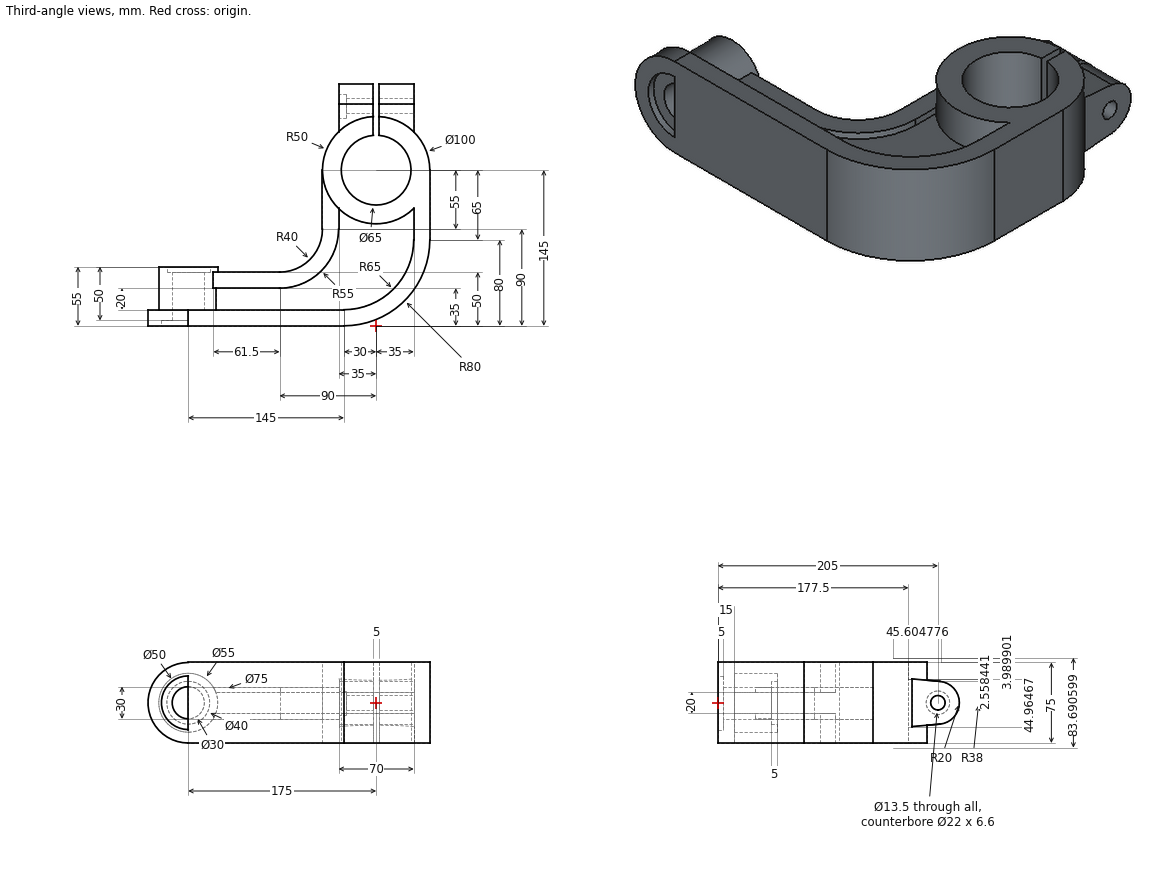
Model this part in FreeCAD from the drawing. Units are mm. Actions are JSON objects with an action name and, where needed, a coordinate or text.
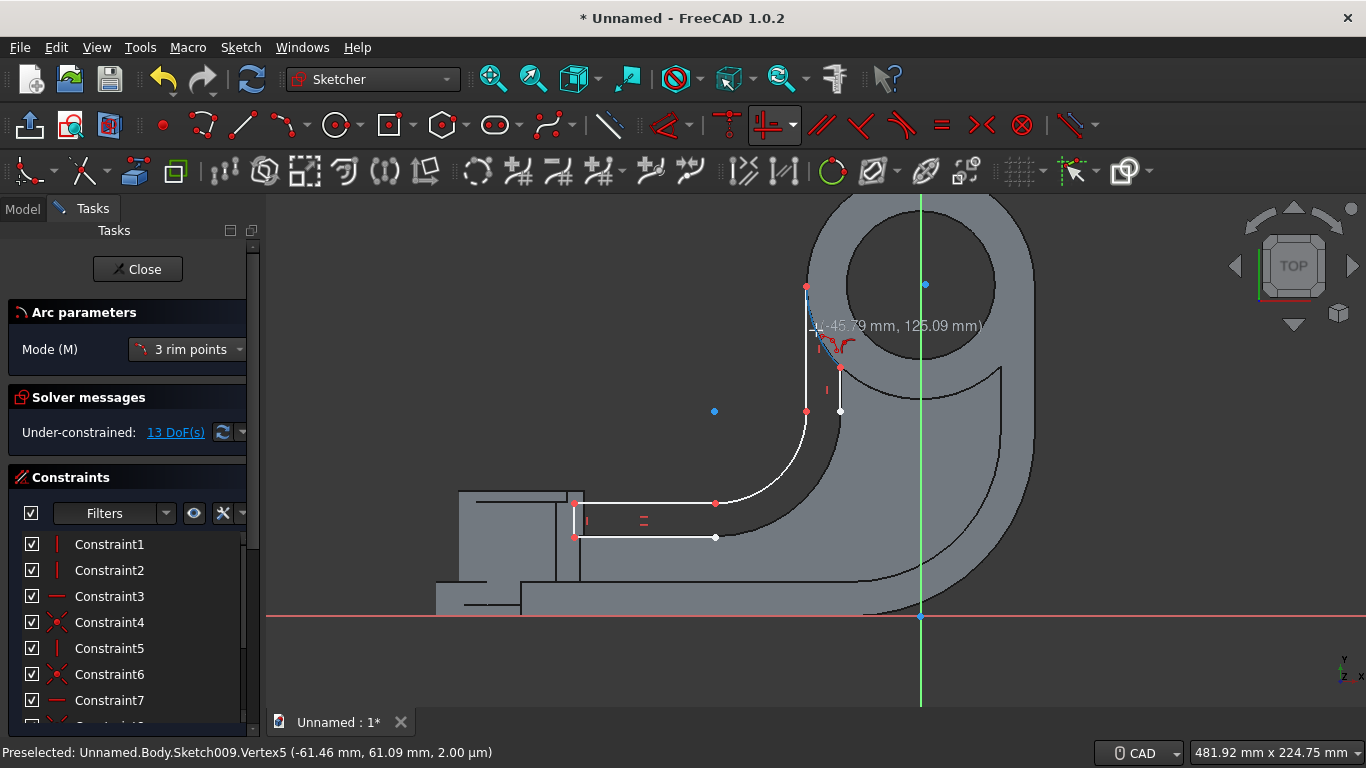
{"action": "left_click", "coordinate": [715, 537]}
{"action": "left_click", "coordinate": [840, 411]}
{"action": "left_click", "coordinate": [804, 500]}
{"action": "key", "text": "Escape"}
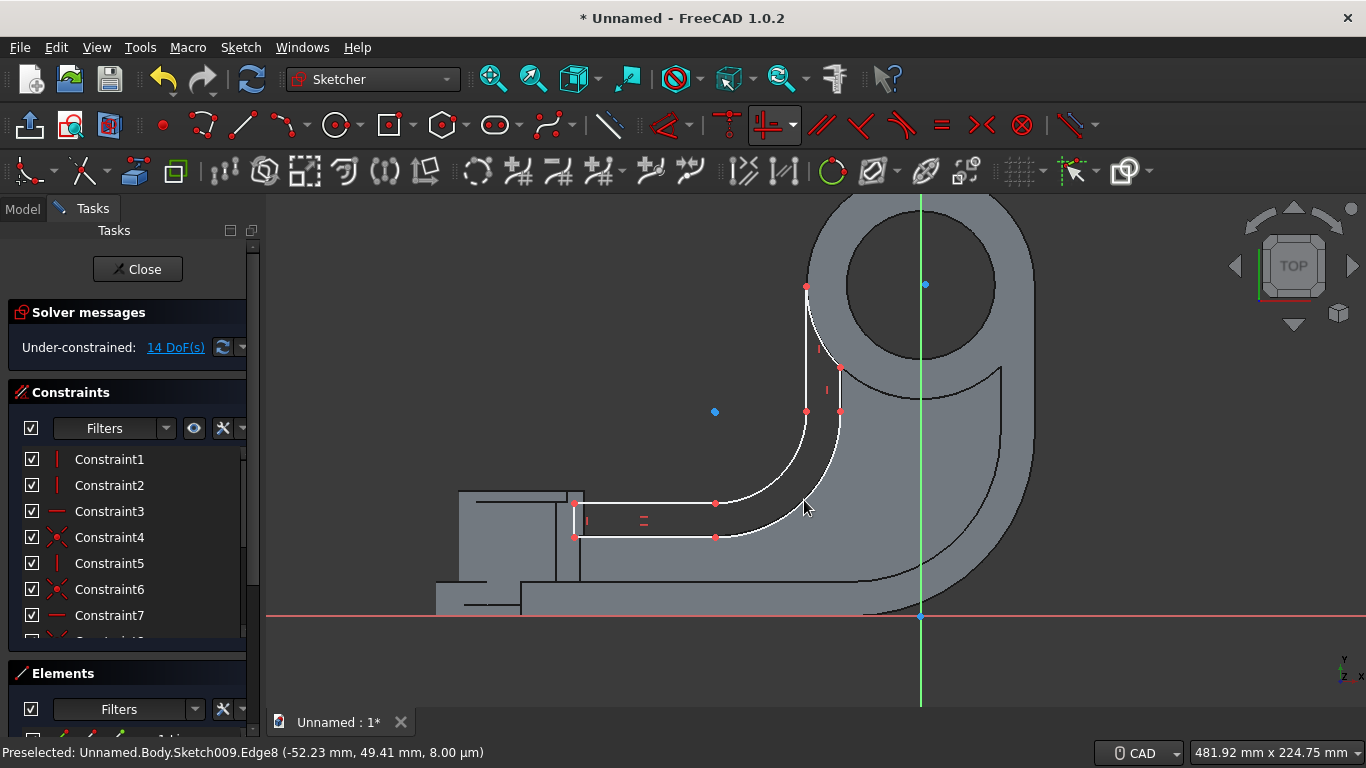
{"action": "left_click", "coordinate": [757, 493]}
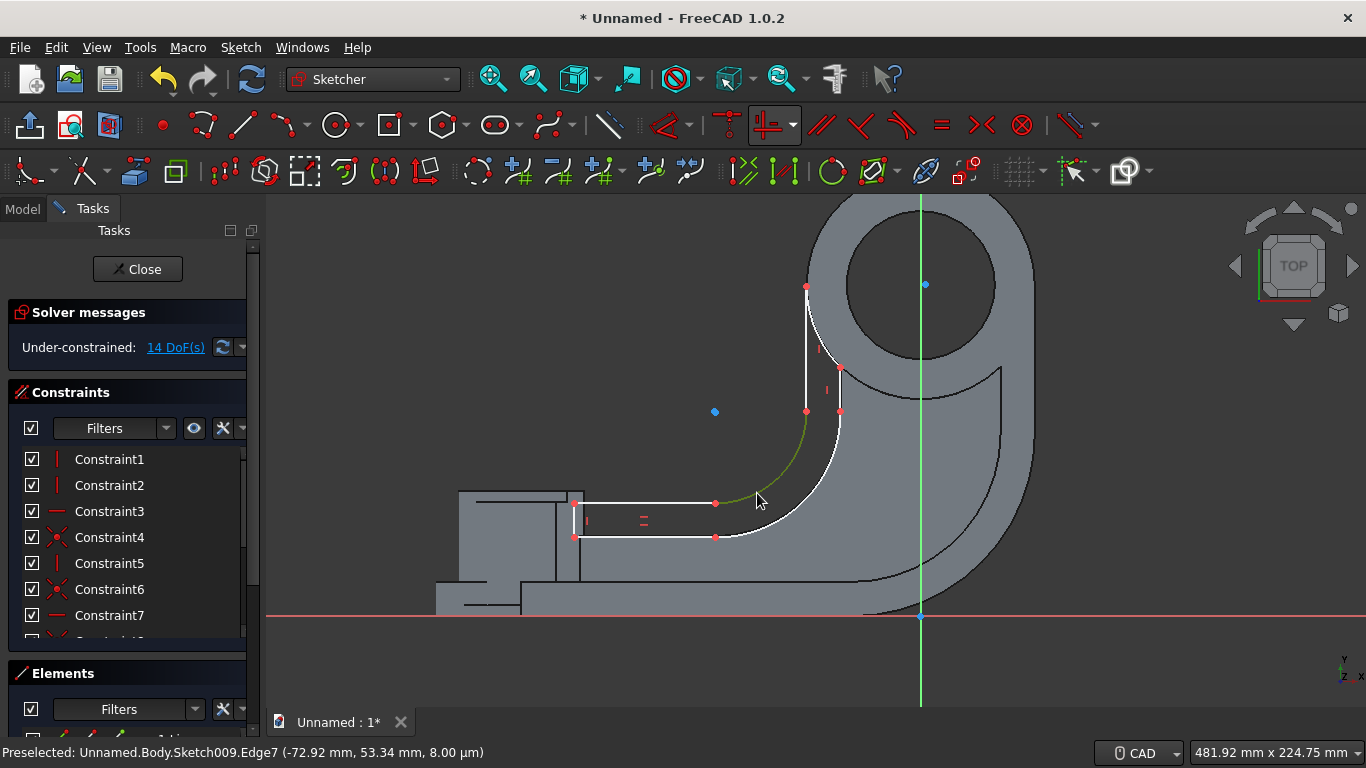
{"action": "left_click", "coordinate": [773, 524]}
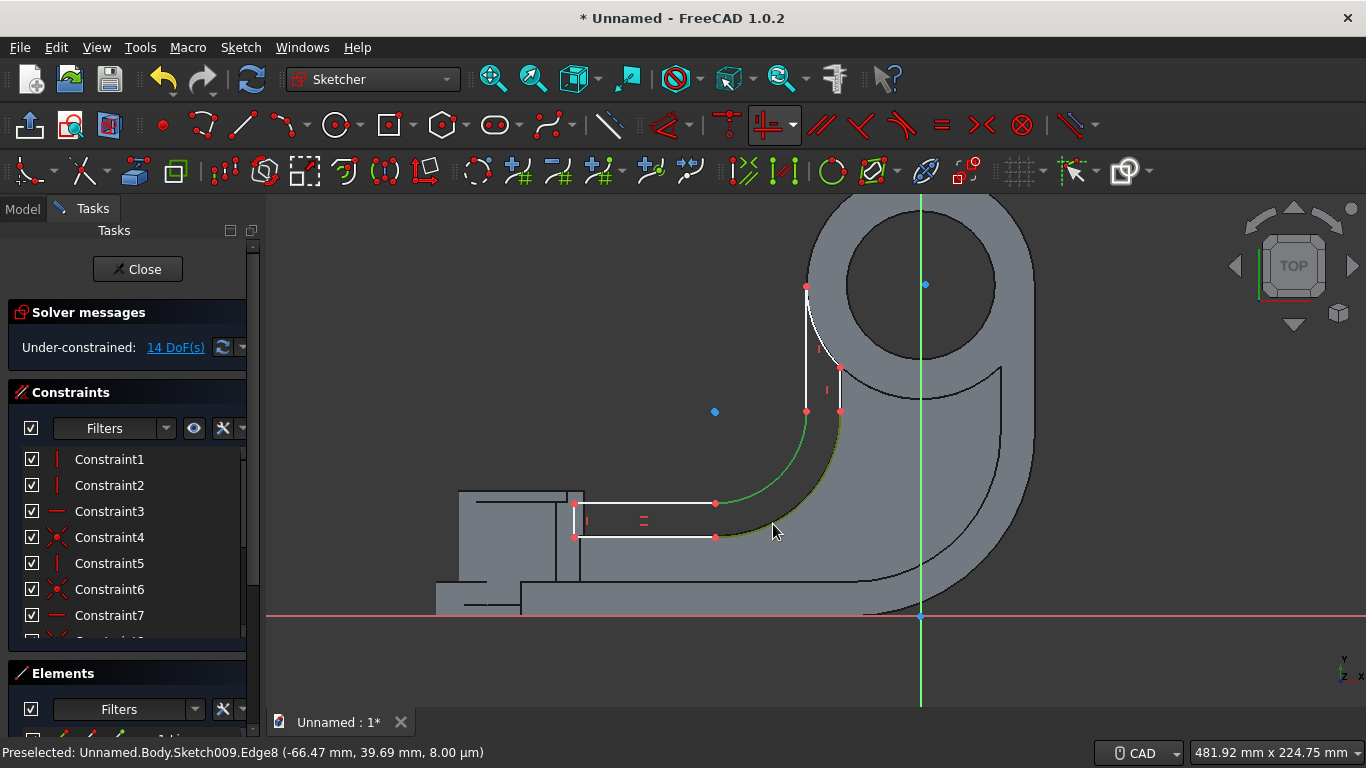
{"action": "left_click", "coordinate": [728, 126]}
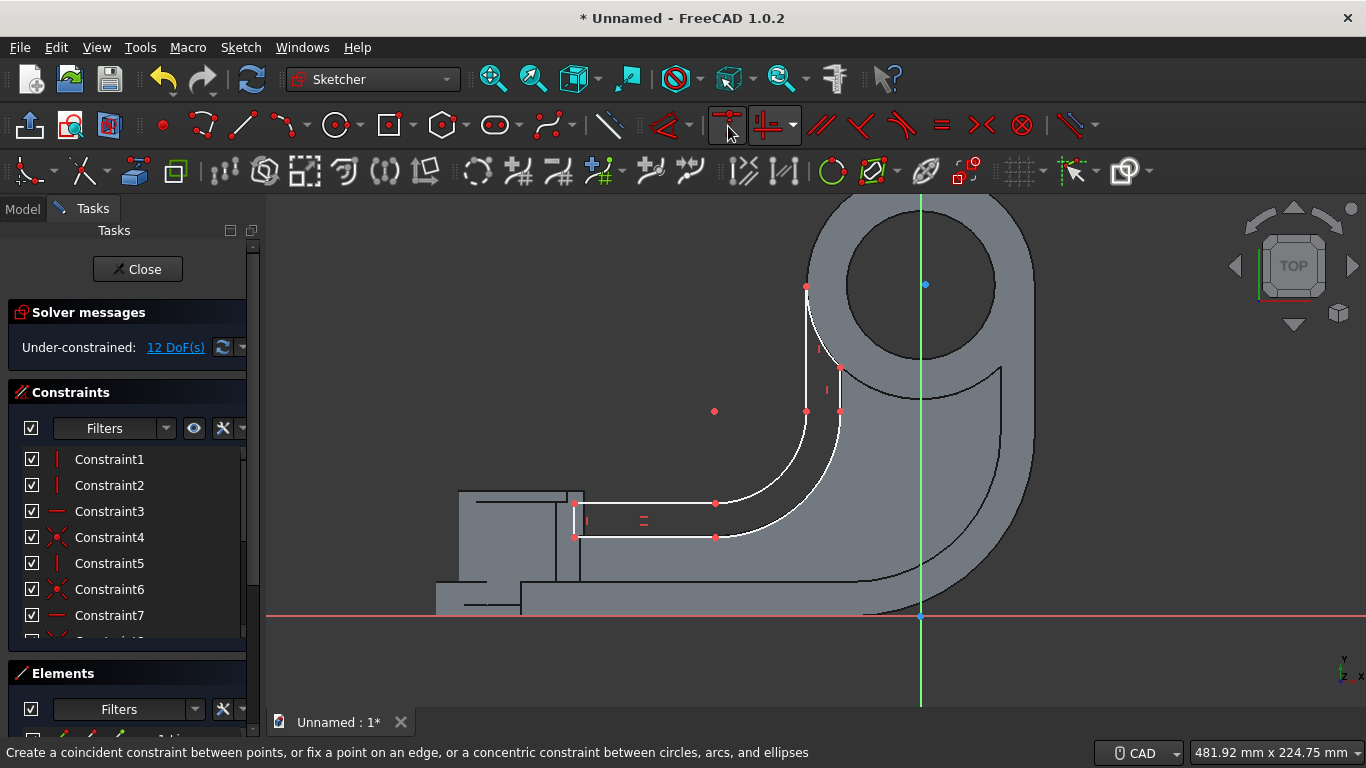
{"action": "left_click", "coordinate": [926, 284]}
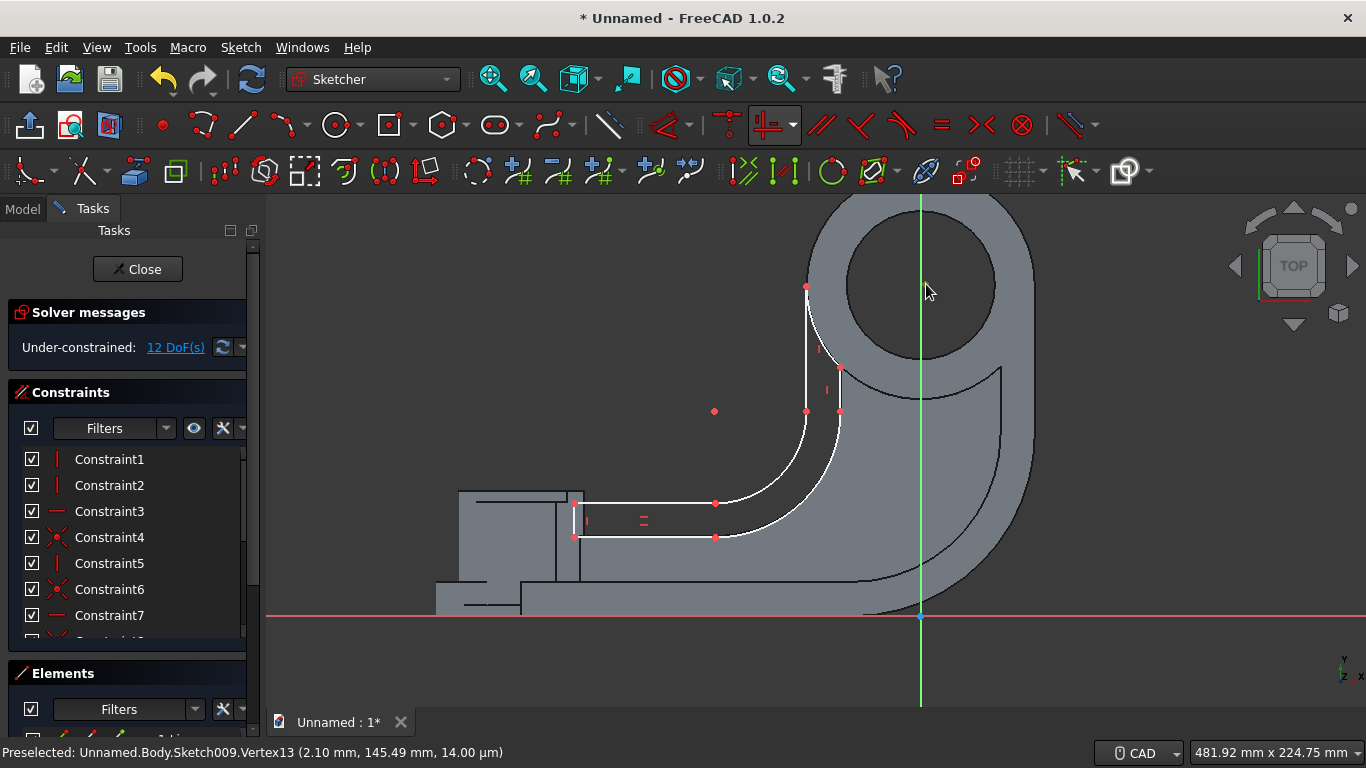
{"action": "left_click", "coordinate": [921, 646]}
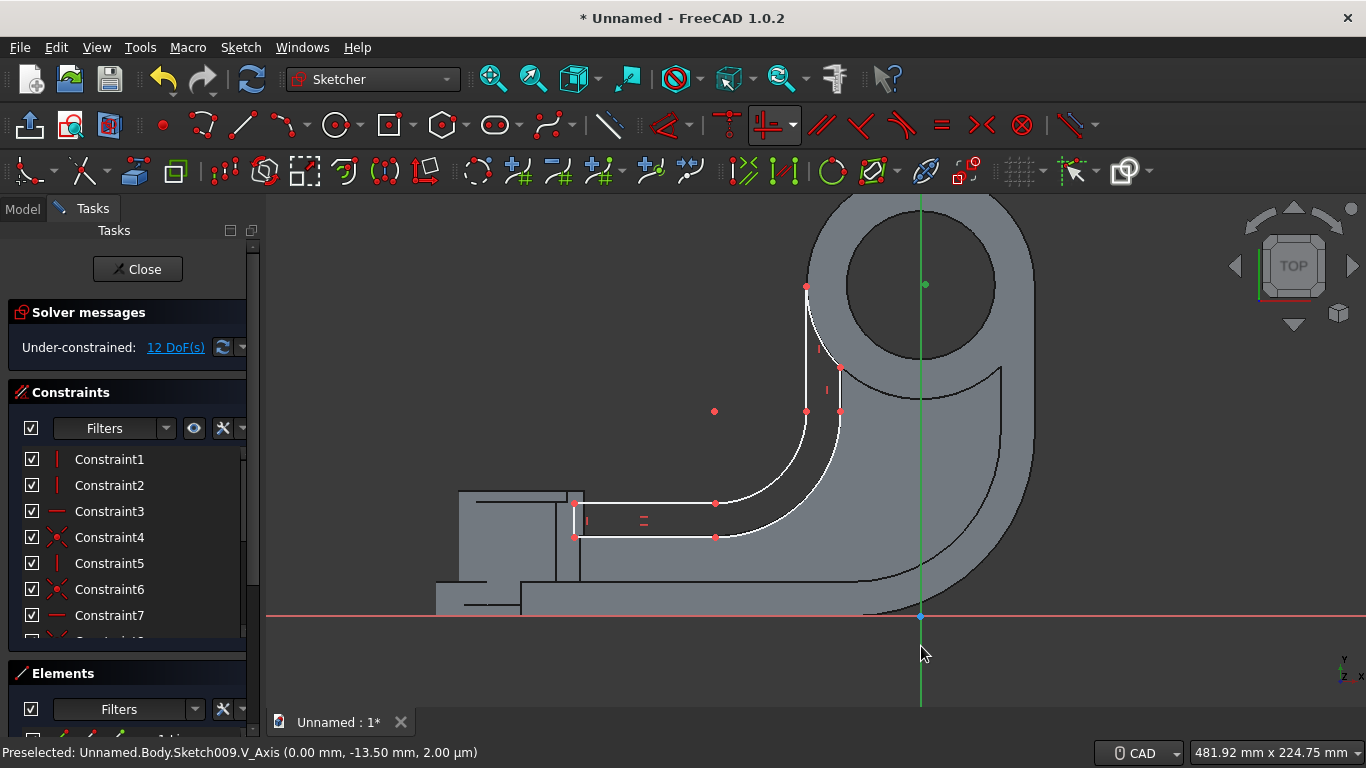
{"action": "key", "text": "c"}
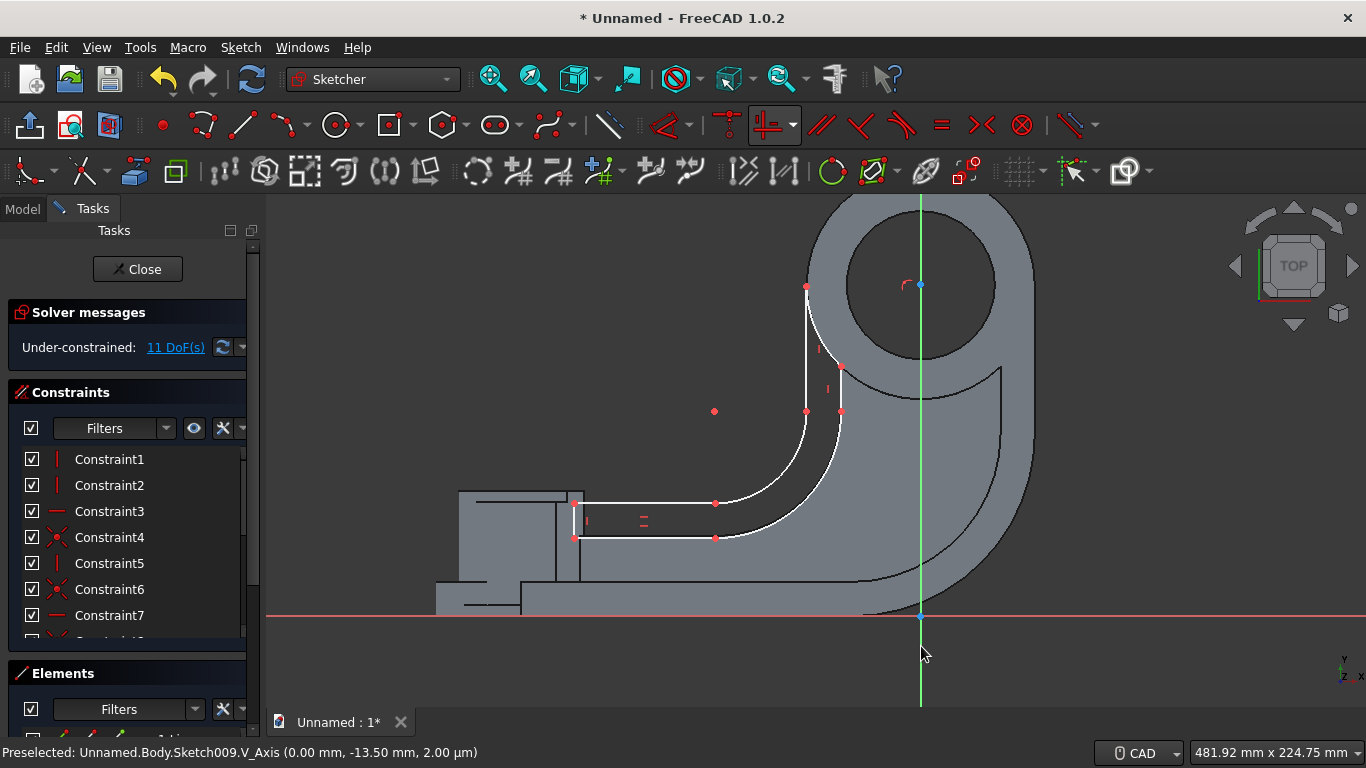
{"action": "key", "text": "d"}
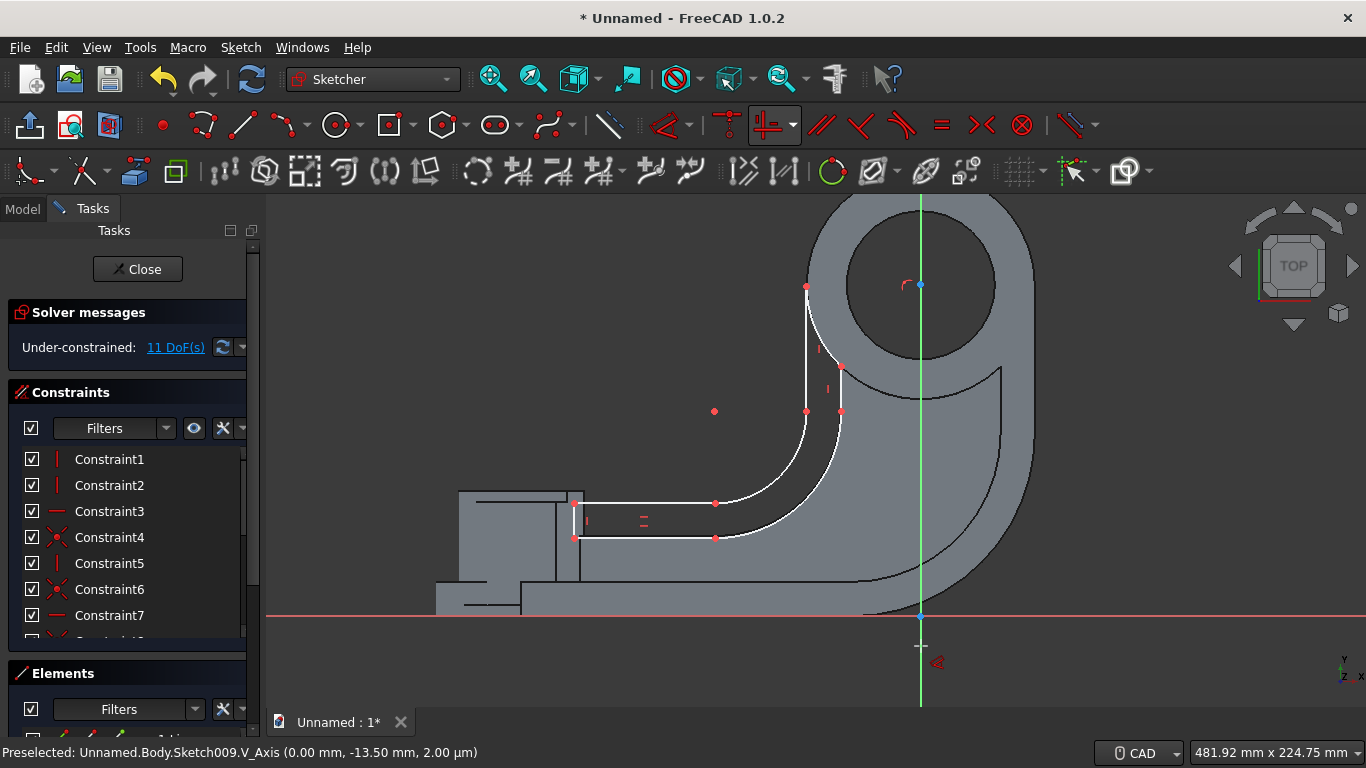
{"action": "left_click", "coordinate": [824, 345]}
{"action": "left_click", "coordinate": [775, 293]}